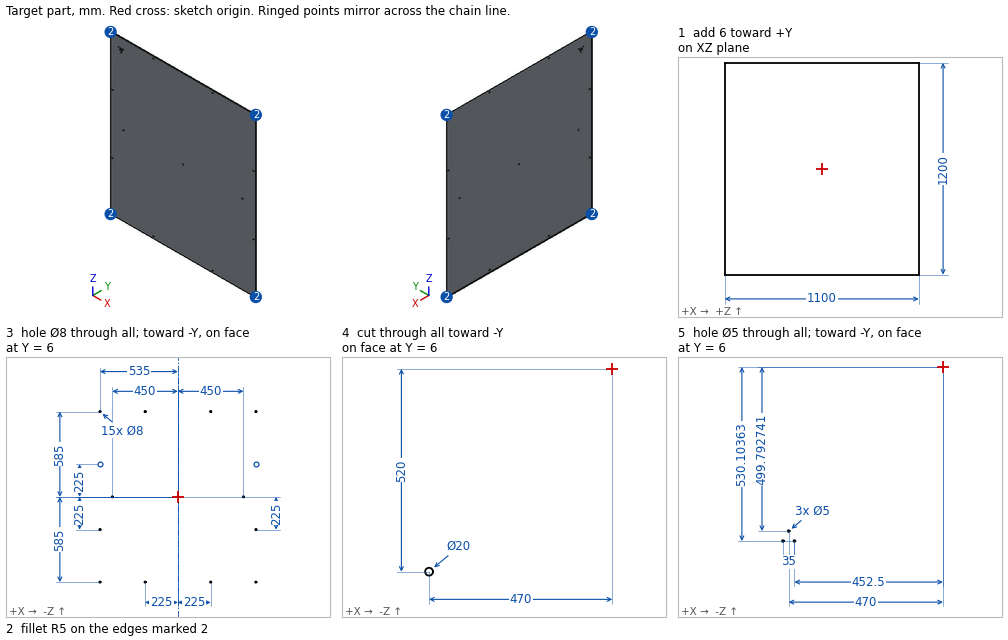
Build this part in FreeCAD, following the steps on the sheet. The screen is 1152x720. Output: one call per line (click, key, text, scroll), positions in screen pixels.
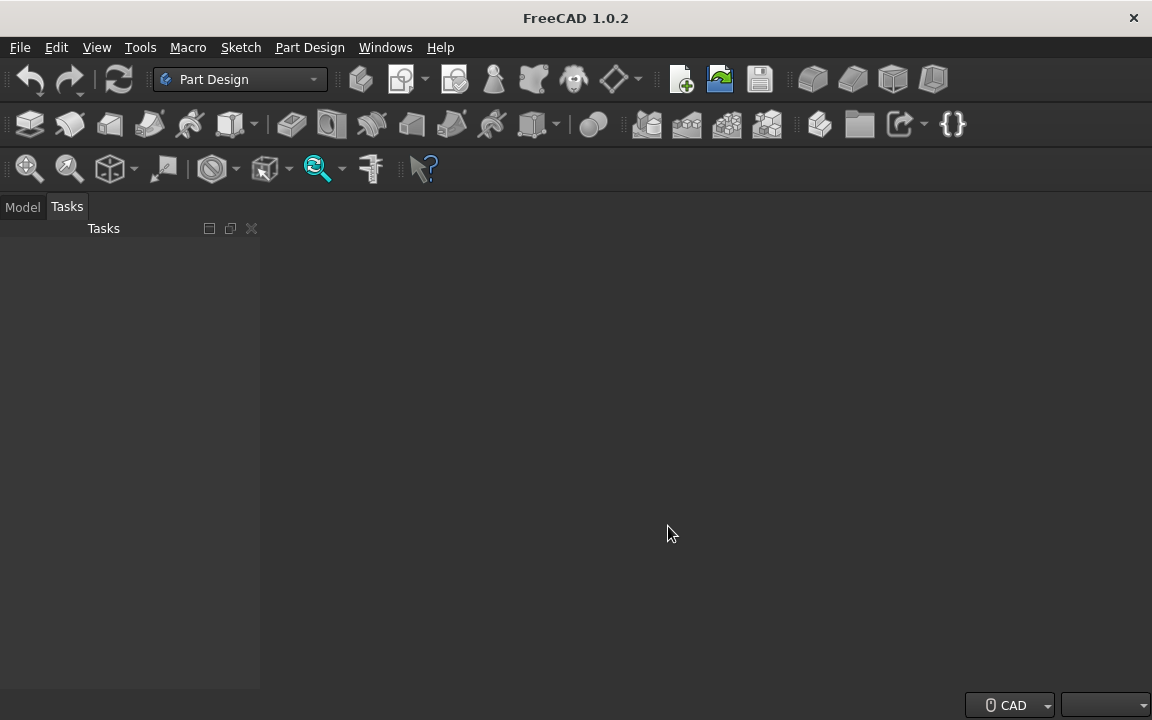
click(680, 80)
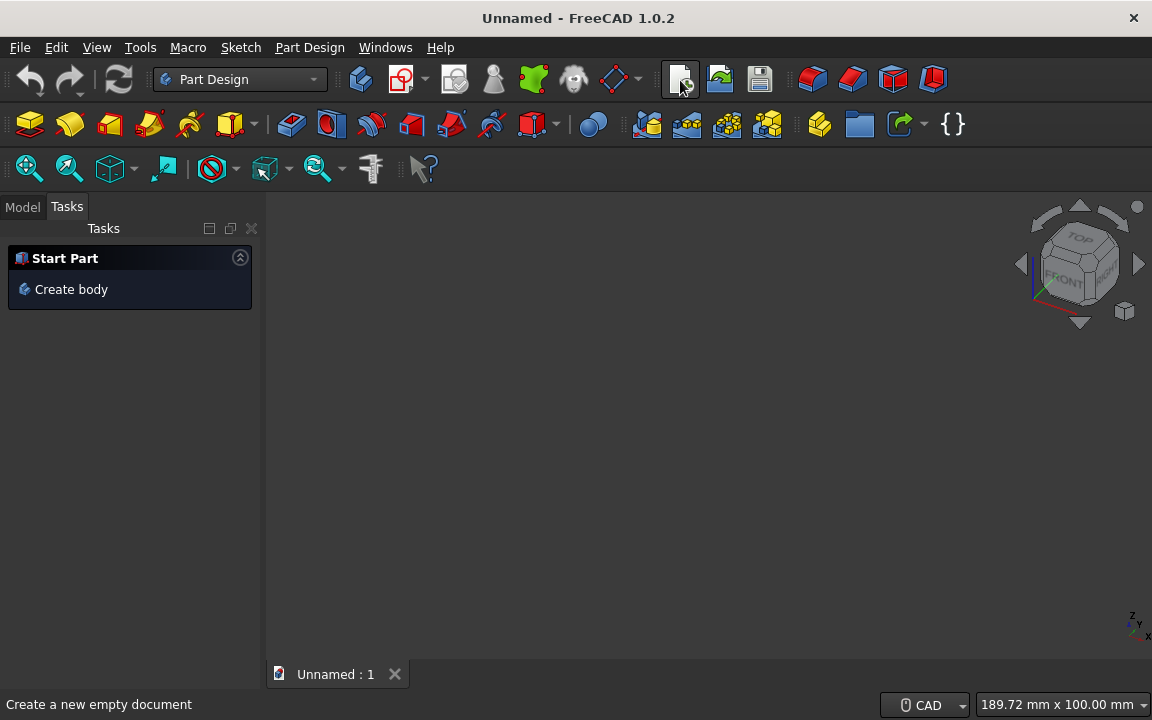
click(402, 80)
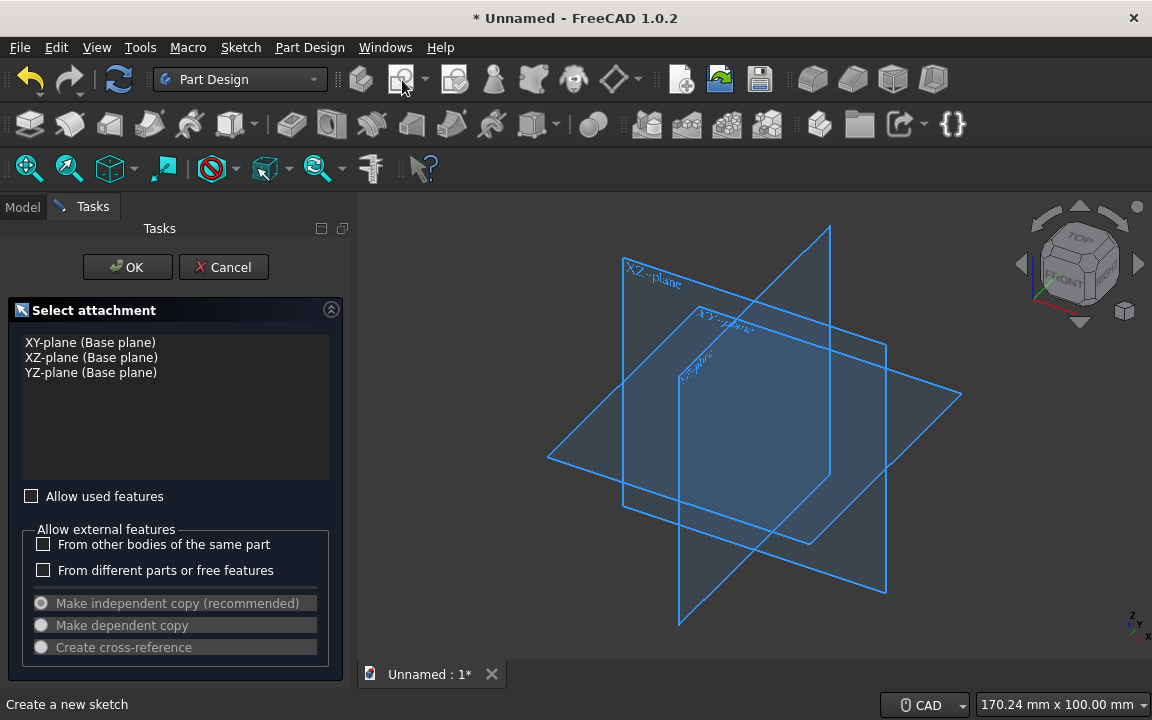
click(82, 358)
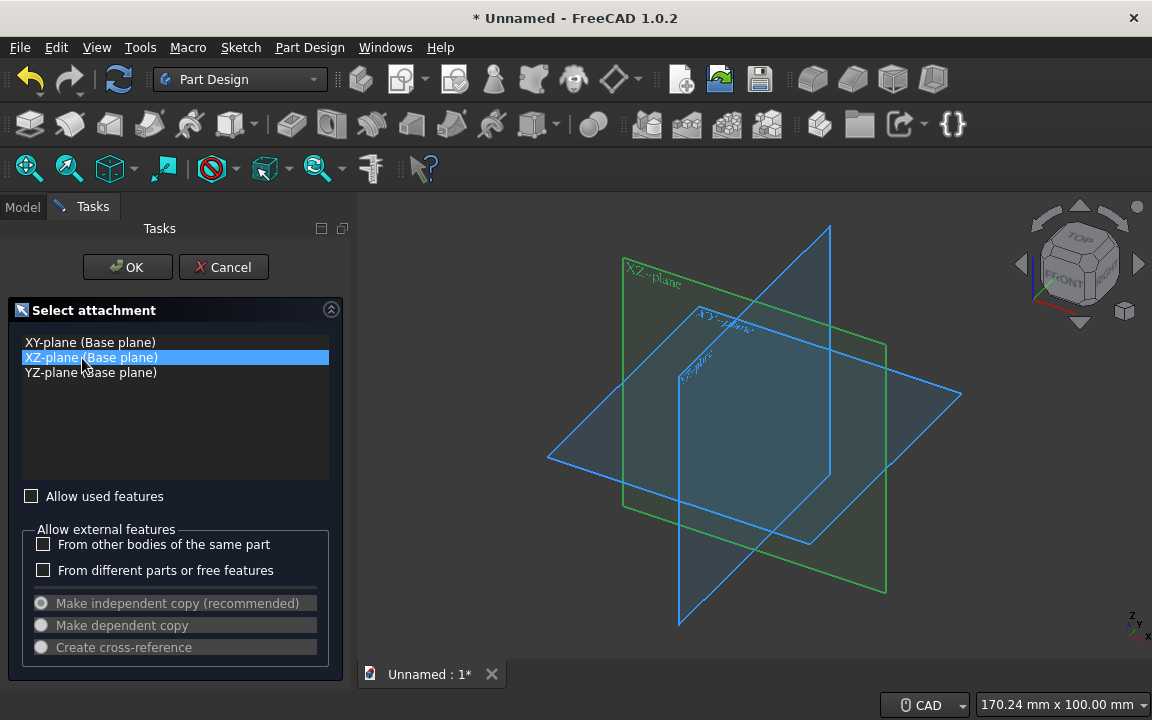
click(128, 267)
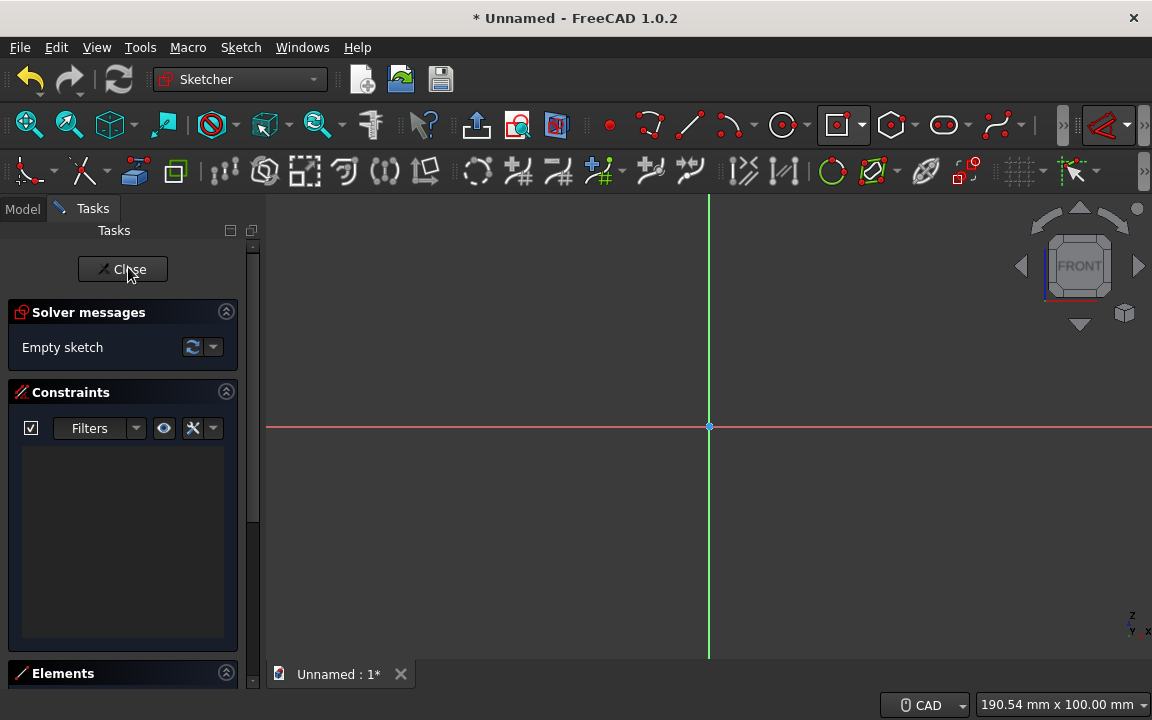
scroll(637, 426, down, 15)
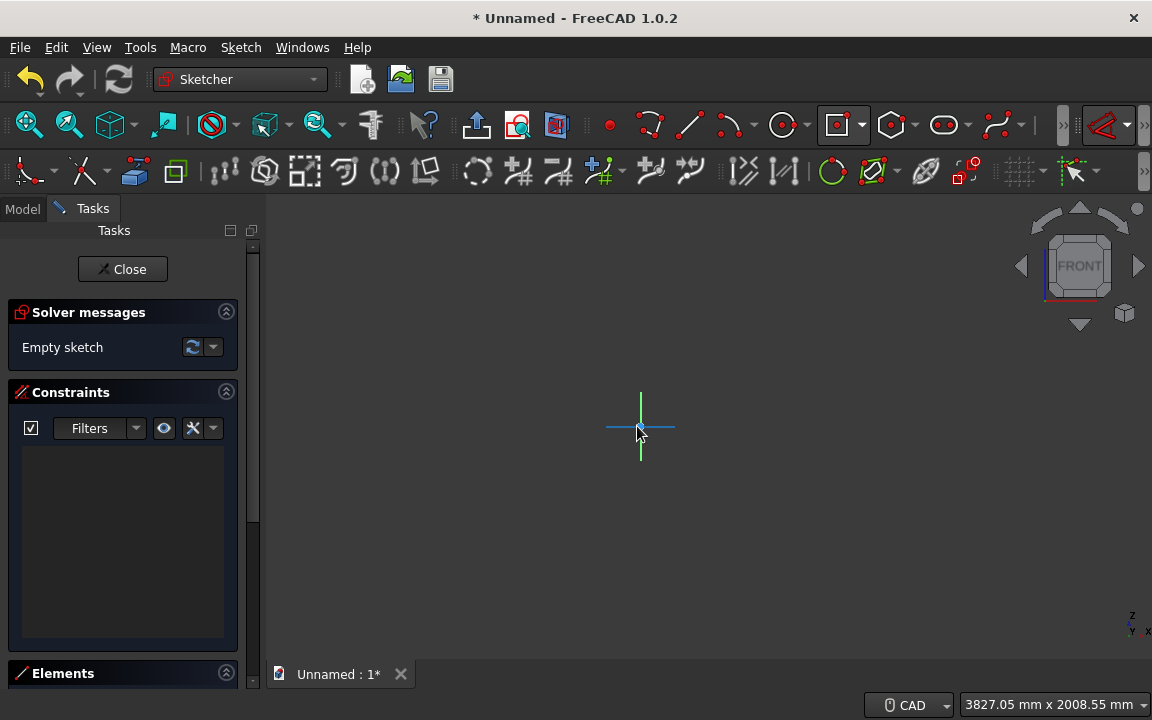
click(838, 126)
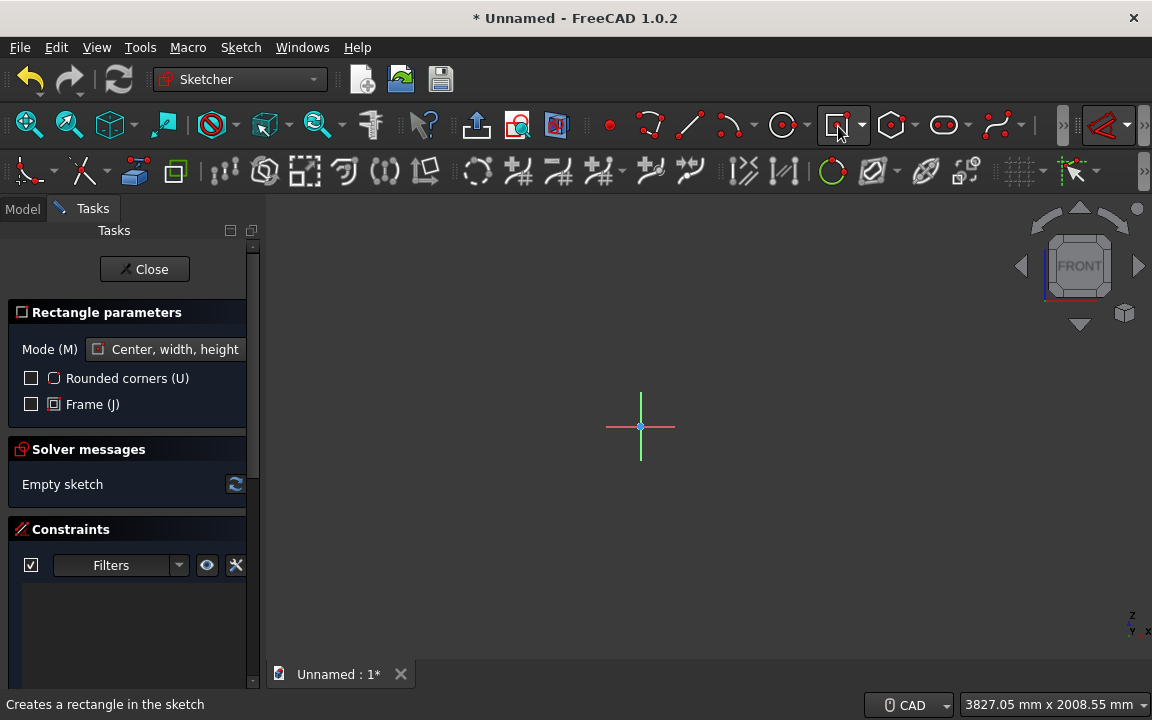
click(641, 426)
move(768, 288)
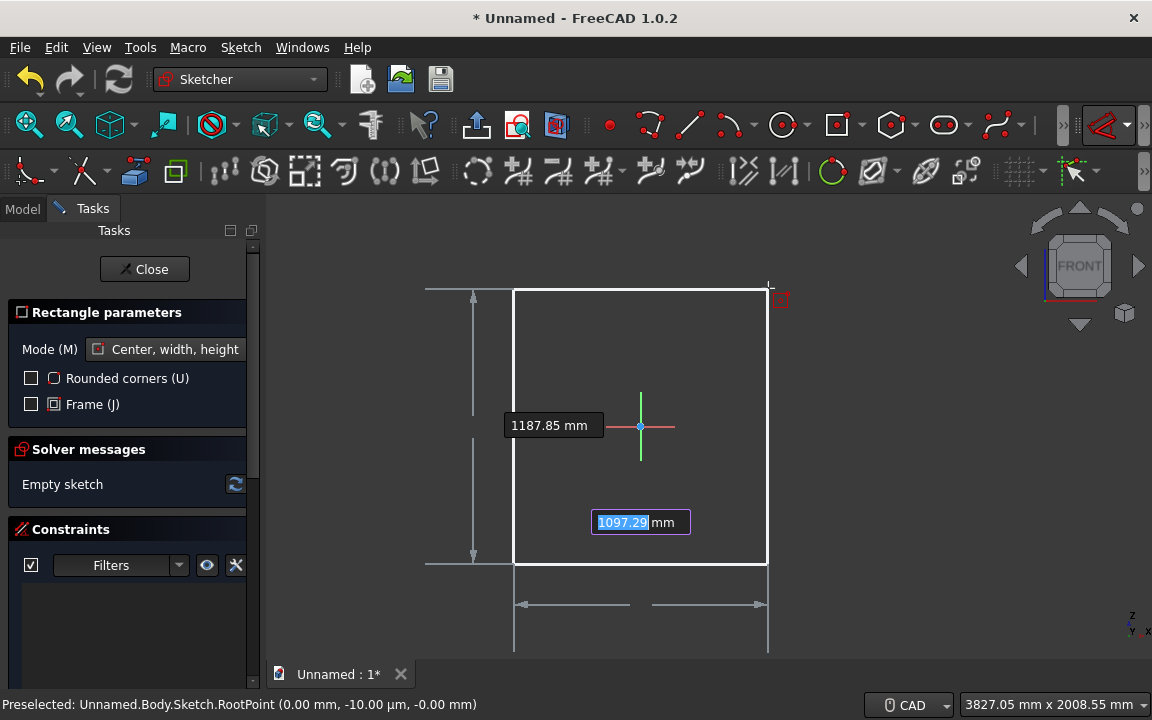
text(1100)
key(Tab)
text(1200)
key(Return)
key(Escape)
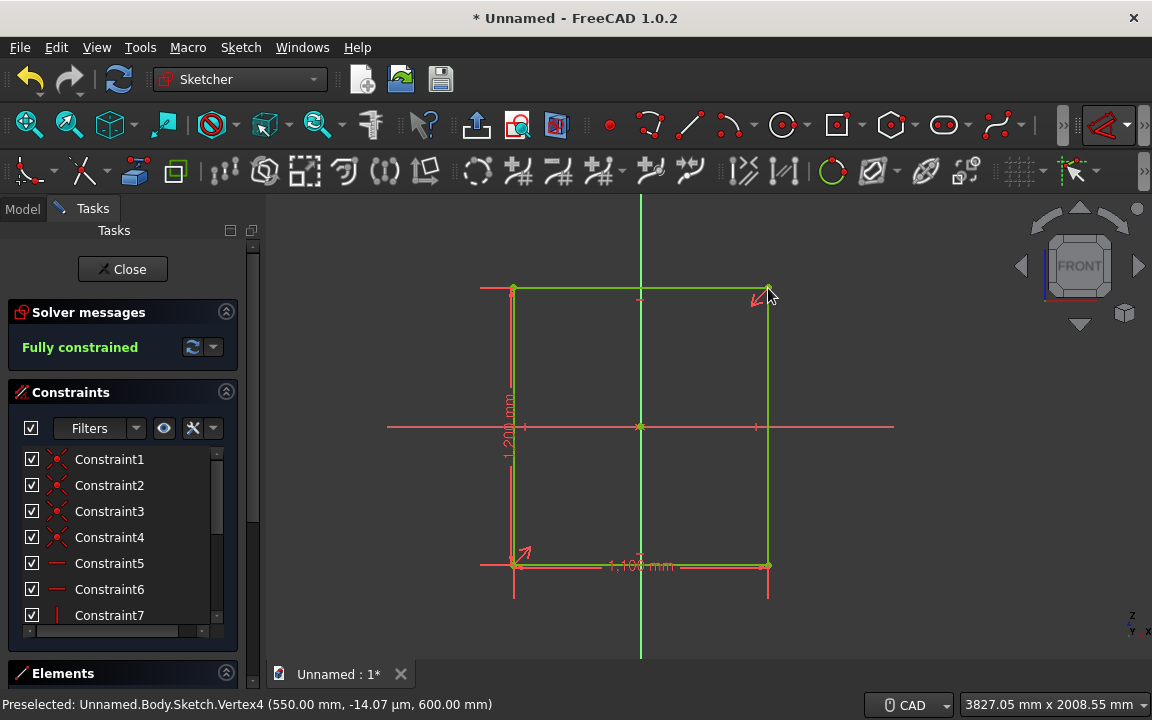
click(123, 269)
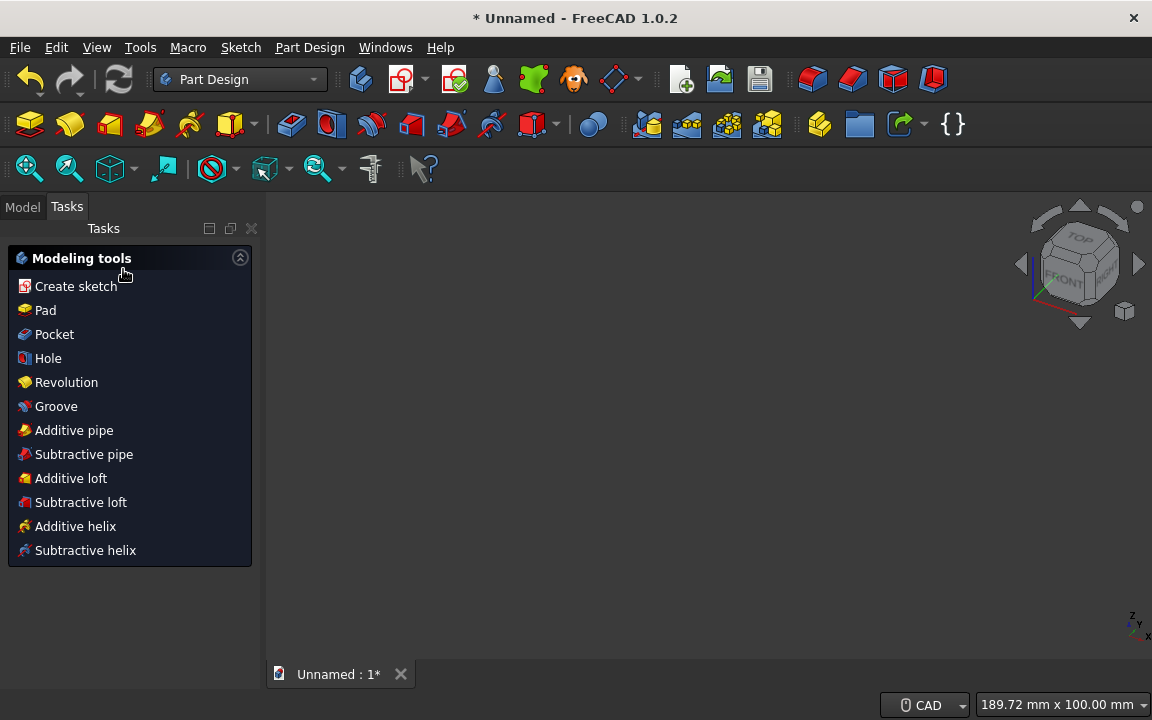
click(30, 124)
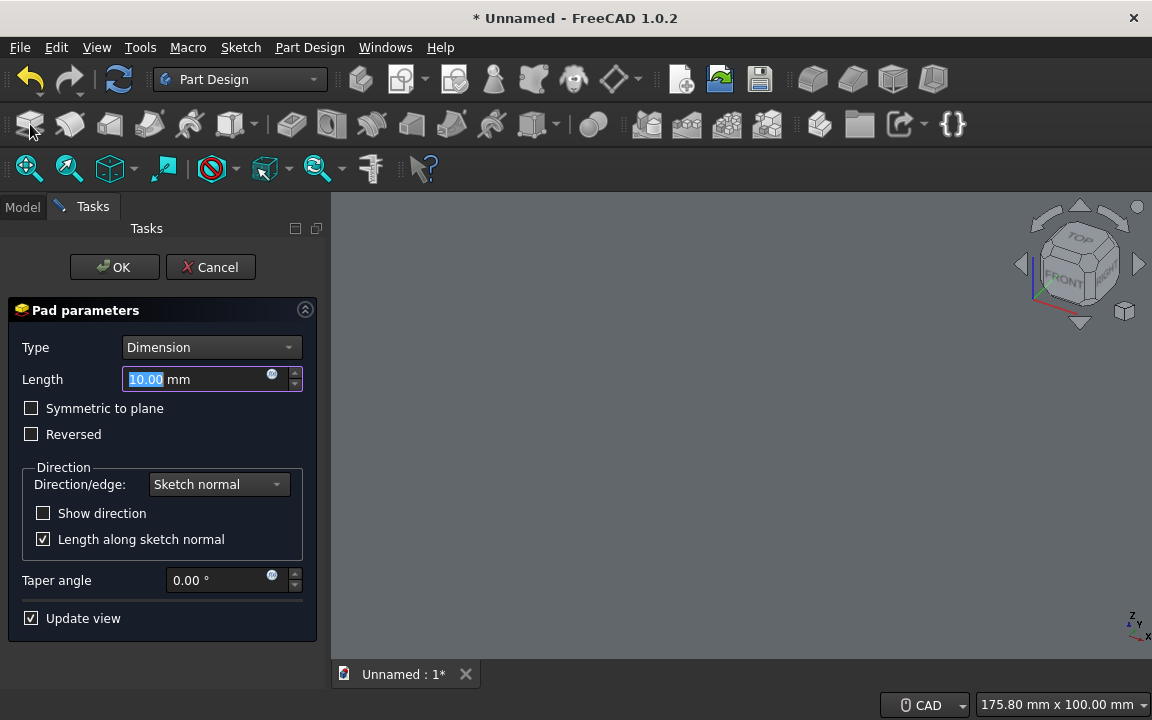
text(6)
key(Tab)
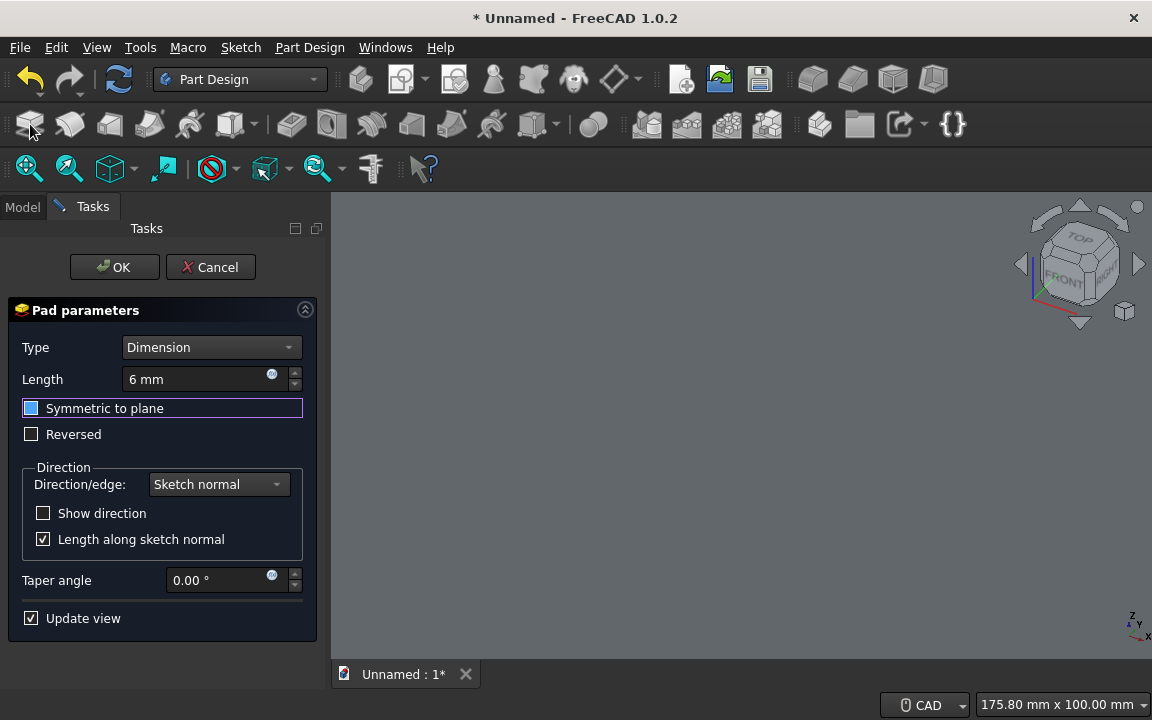
click(30, 434)